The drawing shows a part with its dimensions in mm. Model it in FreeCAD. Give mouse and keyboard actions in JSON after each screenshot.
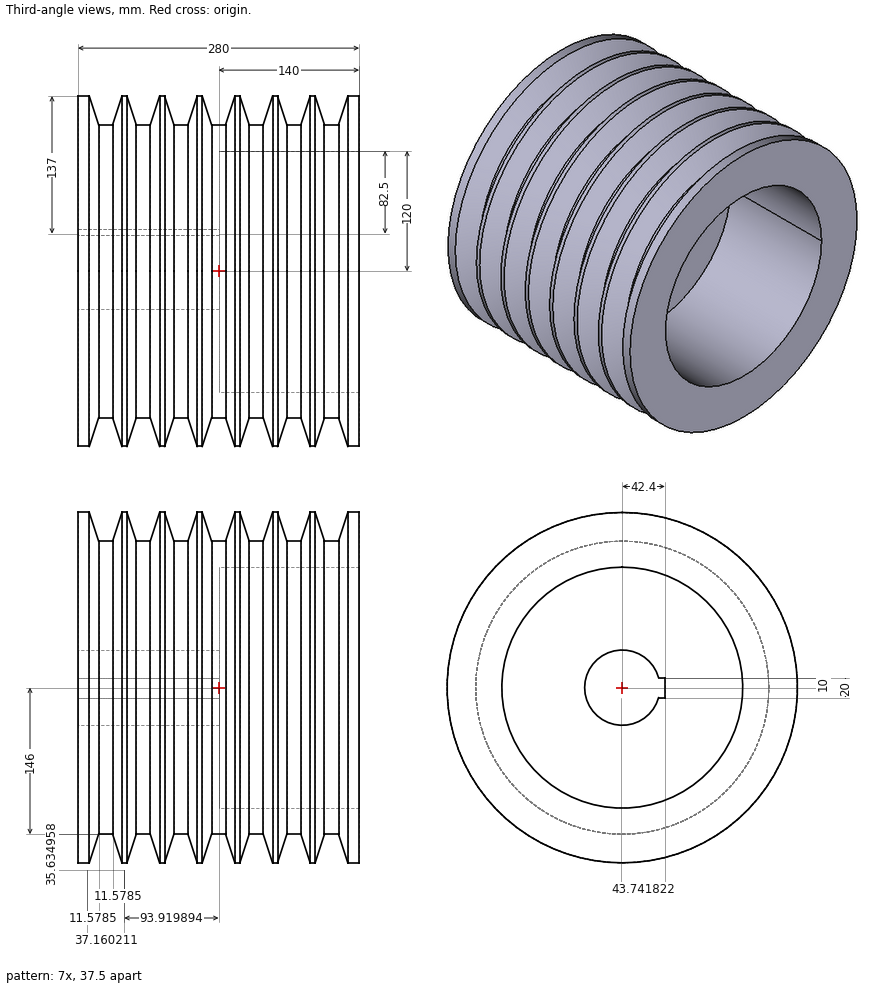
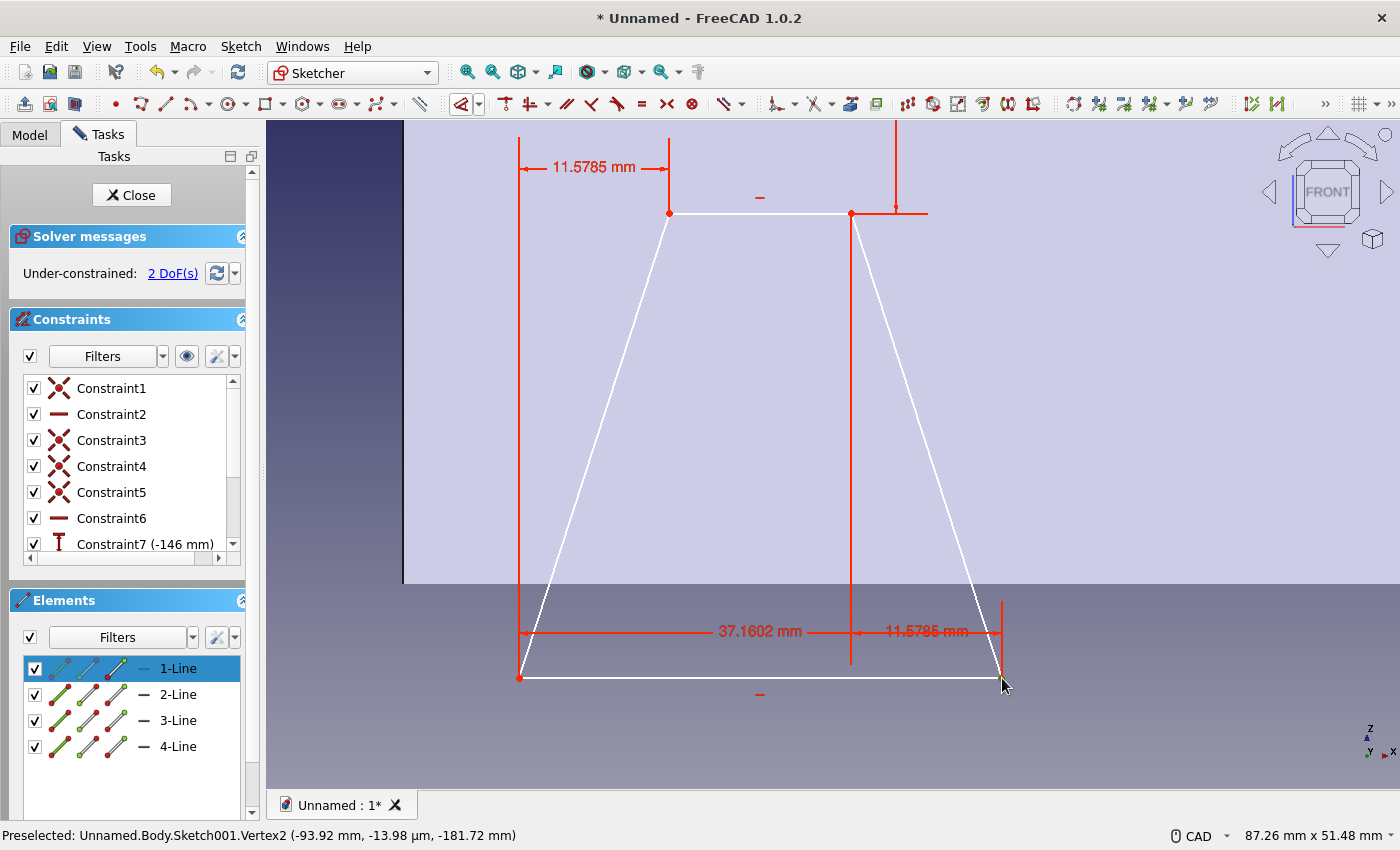
{"action": "key", "text": "l"}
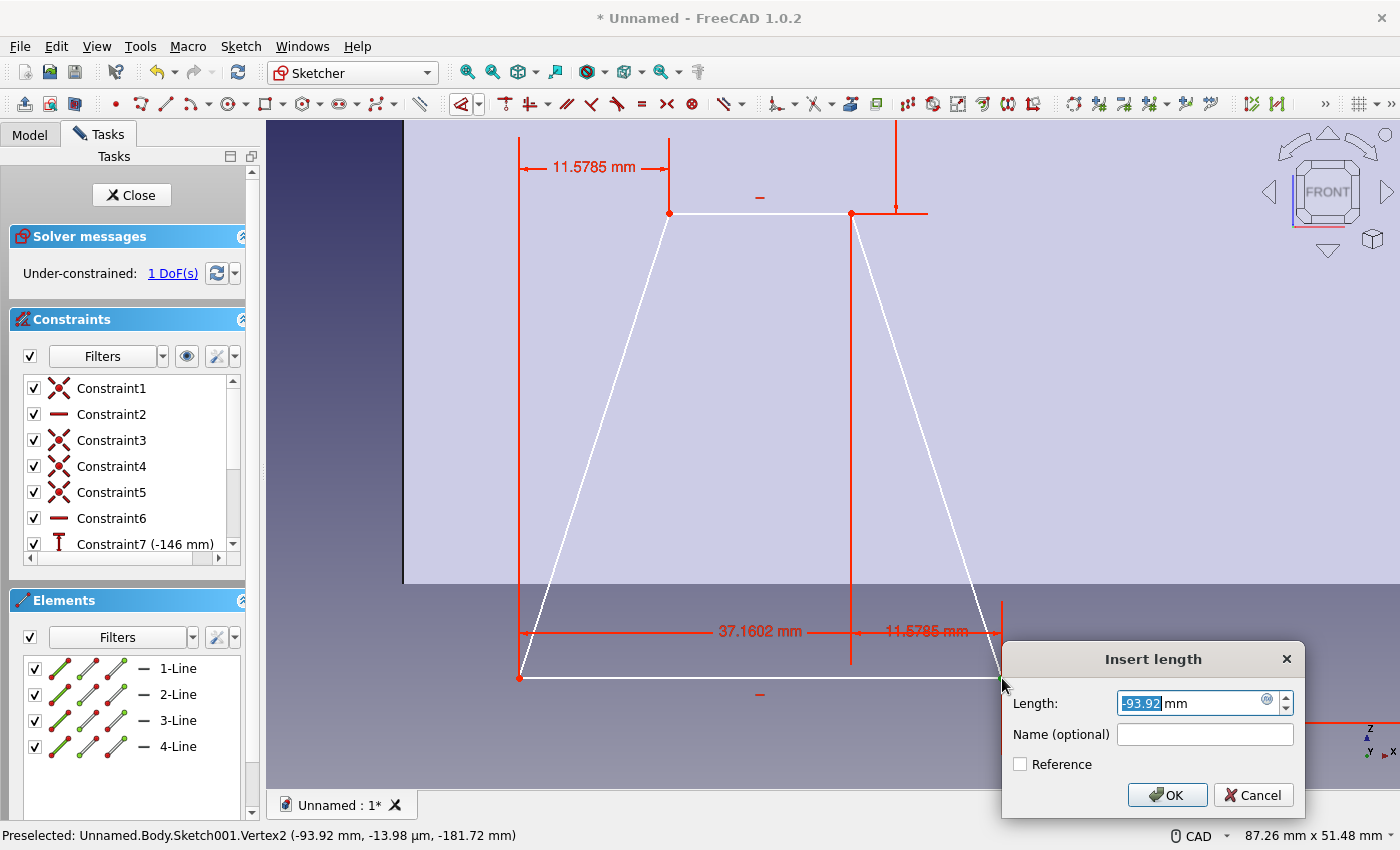
{"action": "type", "text": "-93.919894"}
{"action": "key", "text": "Return"}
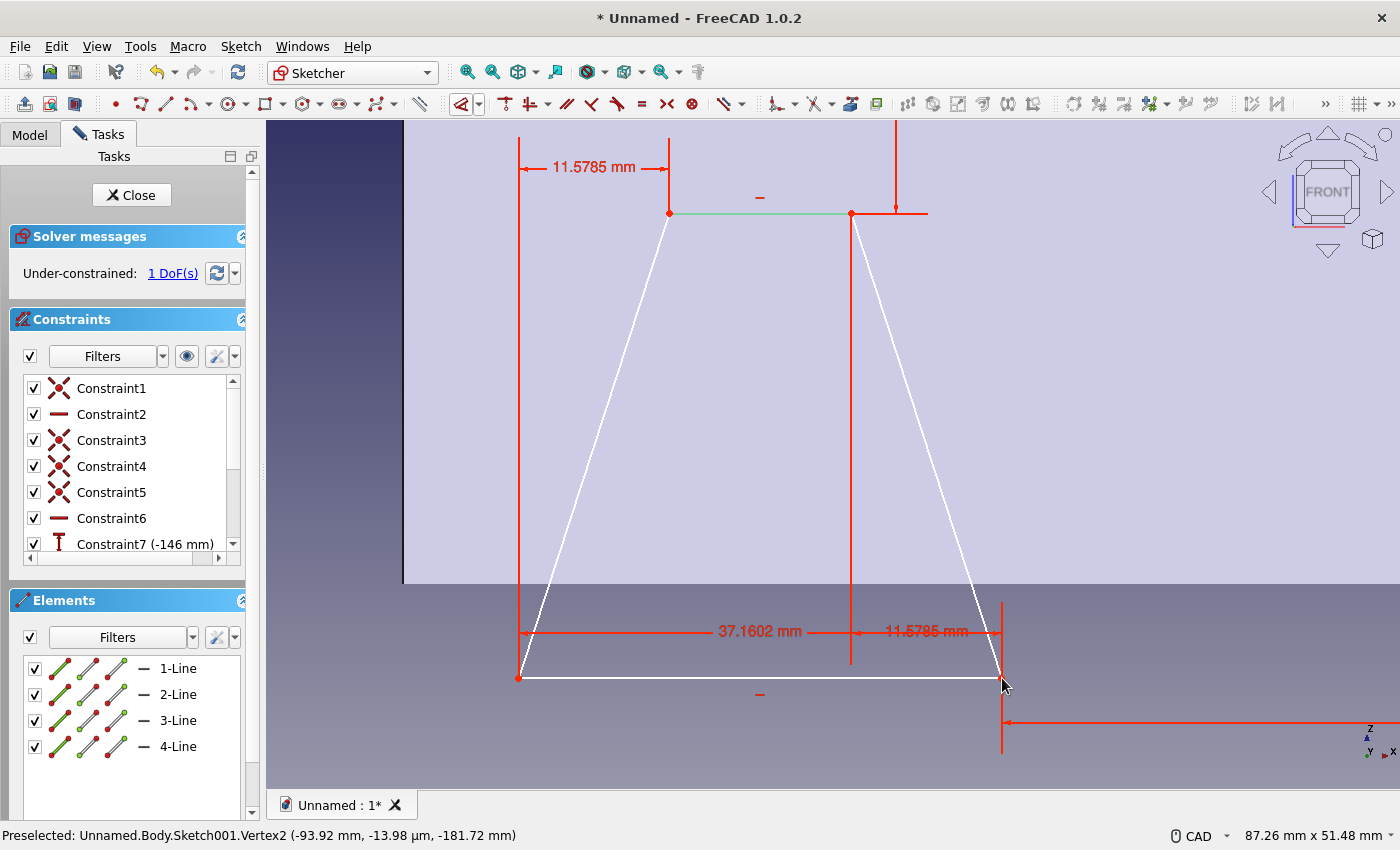
{"action": "left_click", "coordinate": [897, 353]}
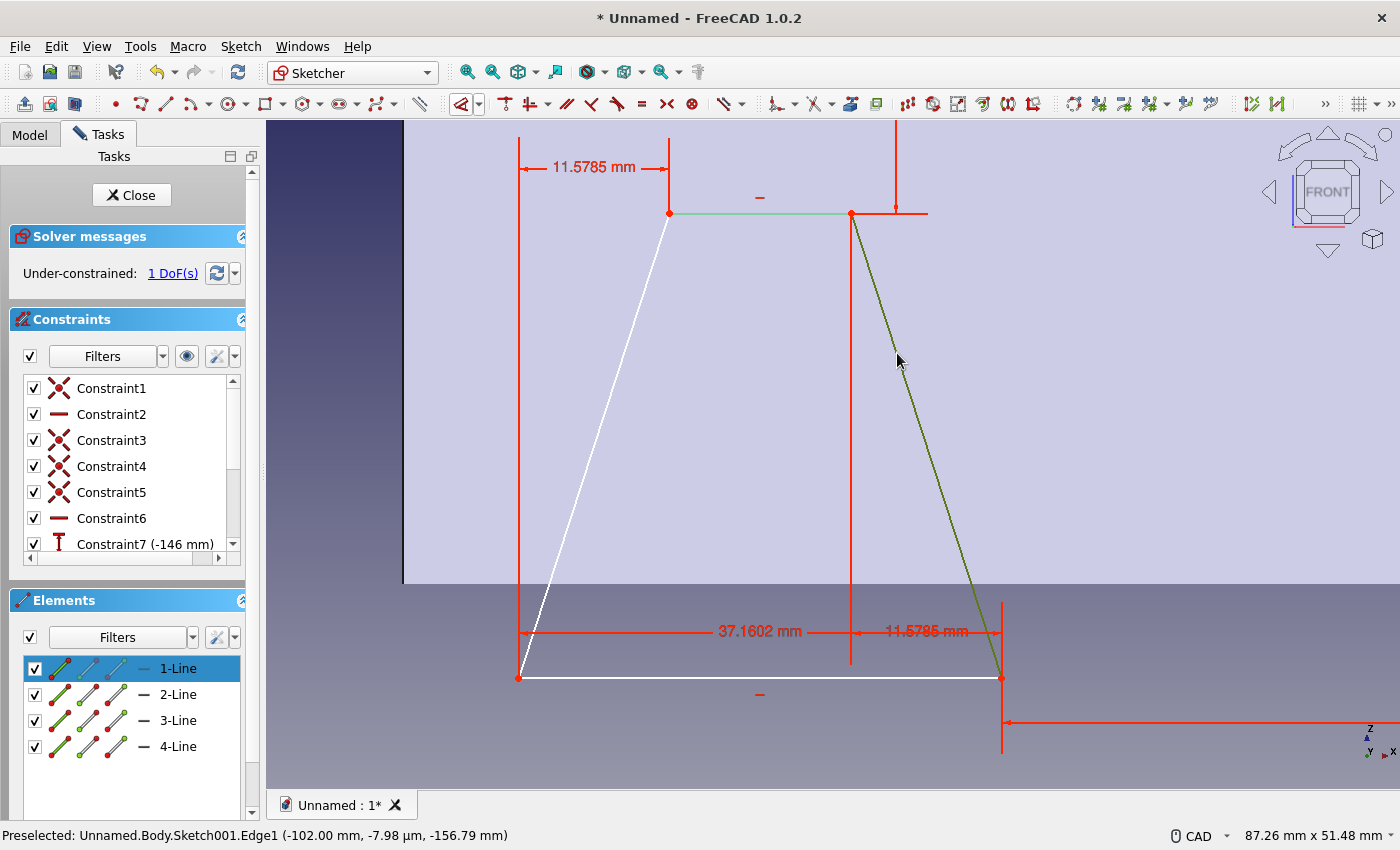
{"action": "left_click", "coordinate": [478, 104]}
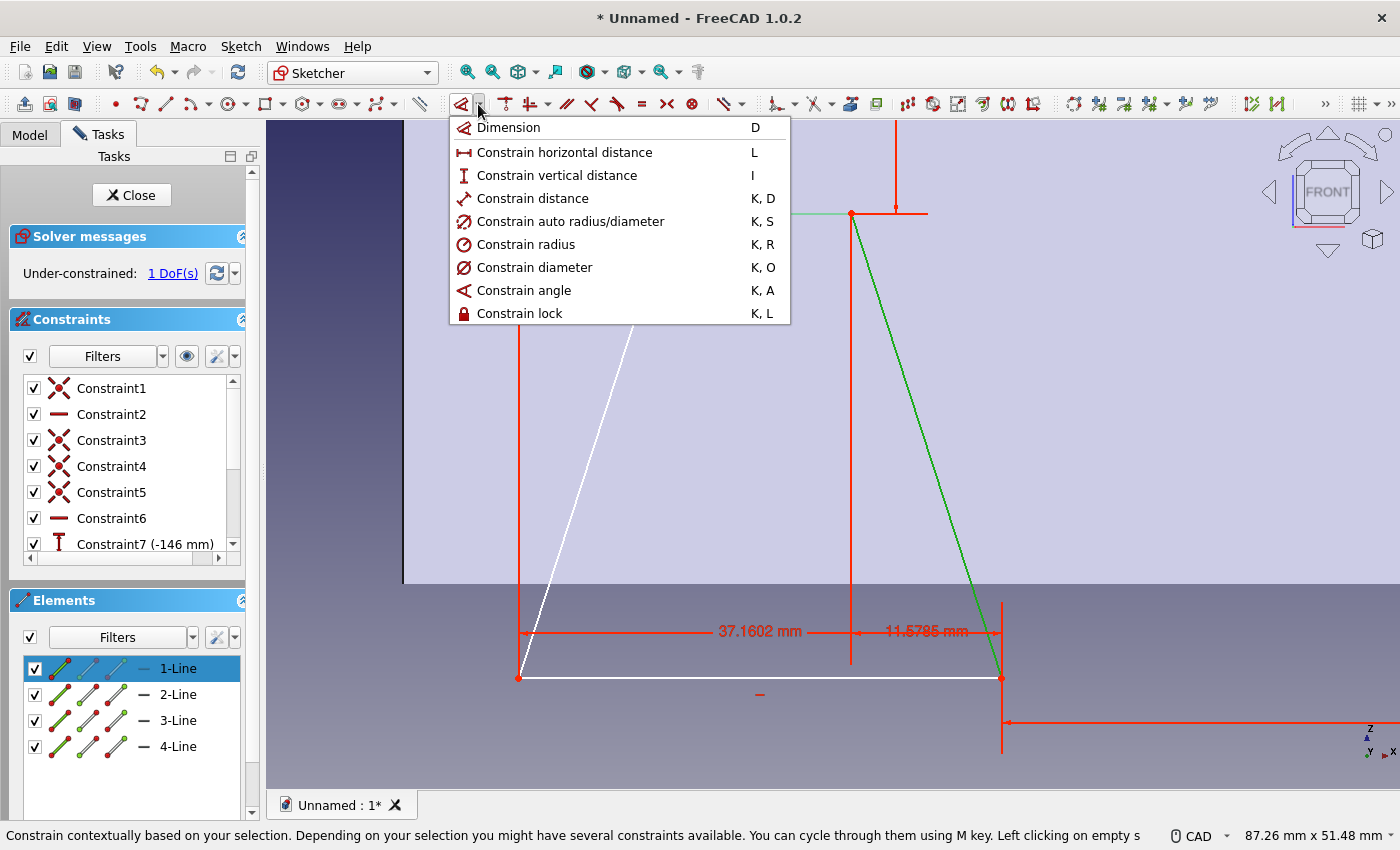
{"action": "left_click", "coordinate": [620, 176]}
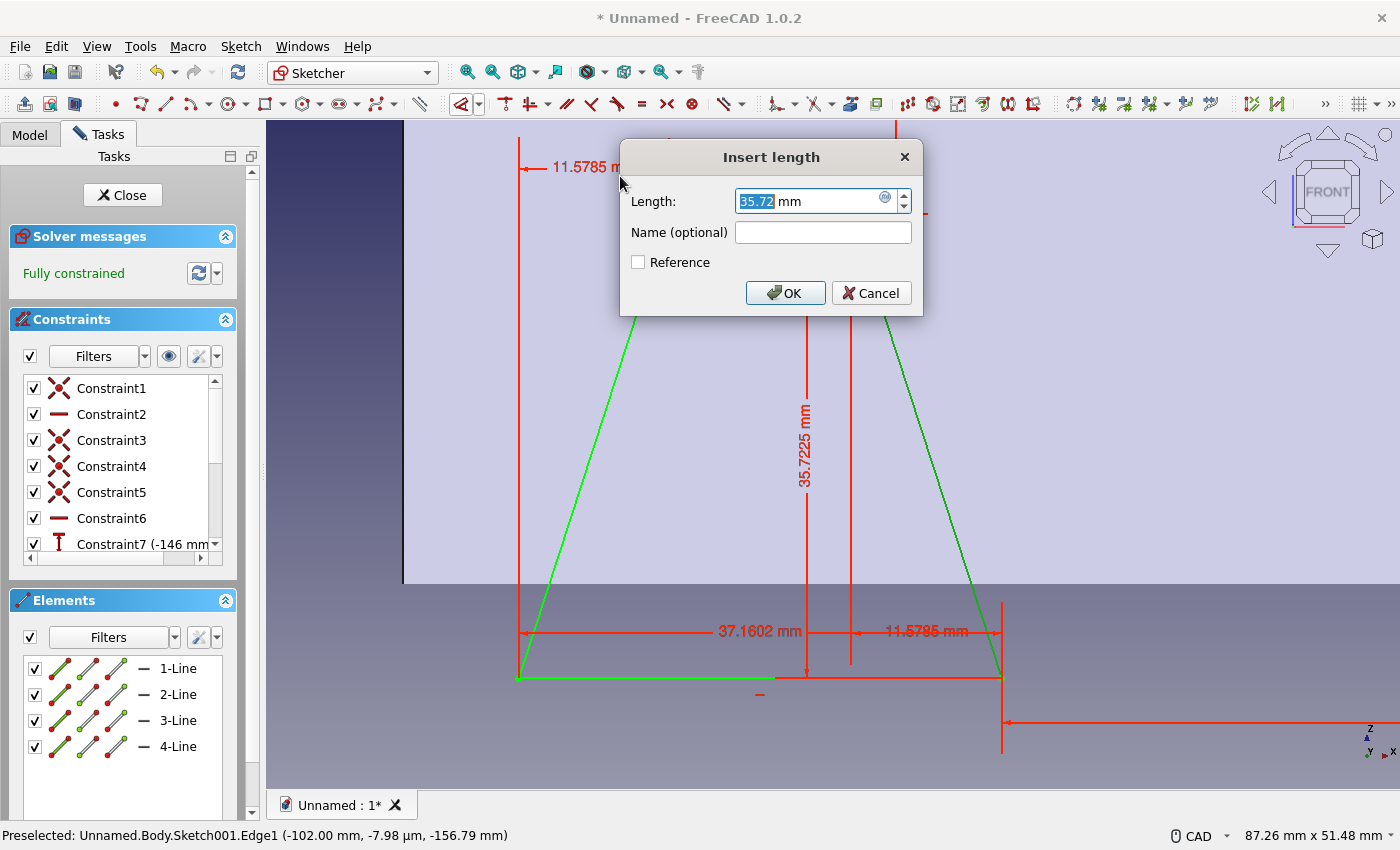
{"action": "type", "text": "35.634958"}
{"action": "key", "text": "Return"}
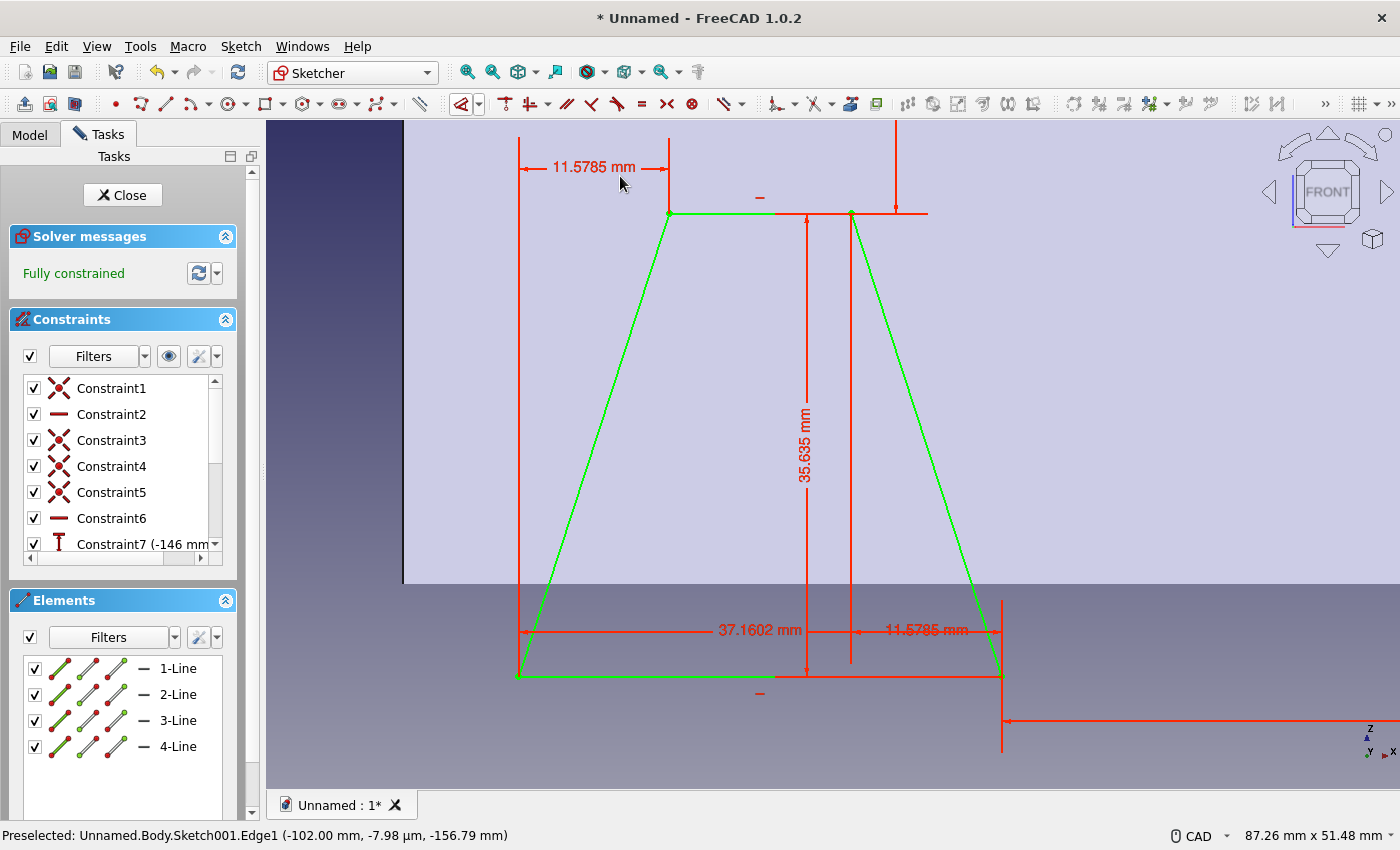
{"action": "left_click", "coordinate": [123, 195]}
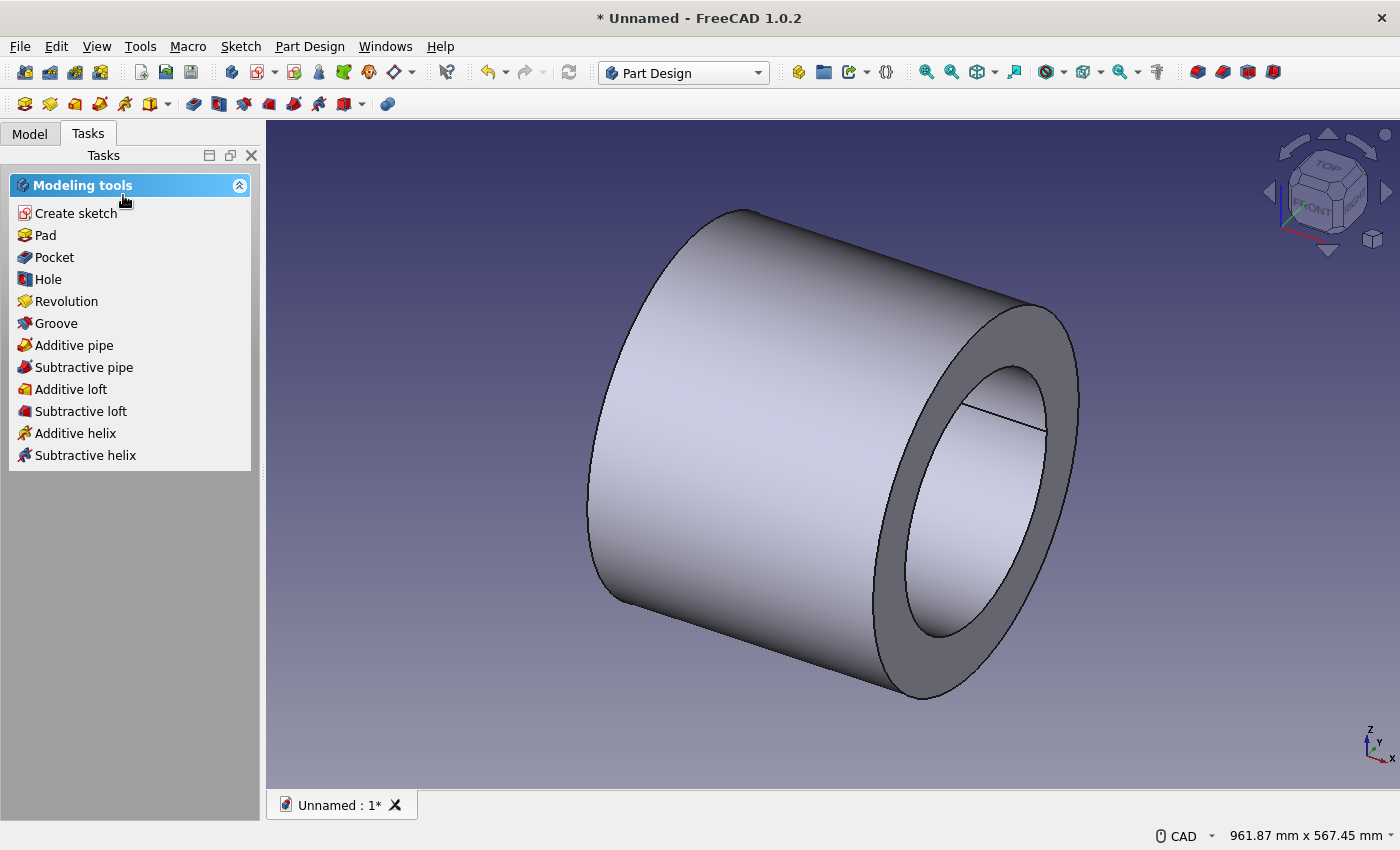
{"action": "left_click", "coordinate": [244, 104]}